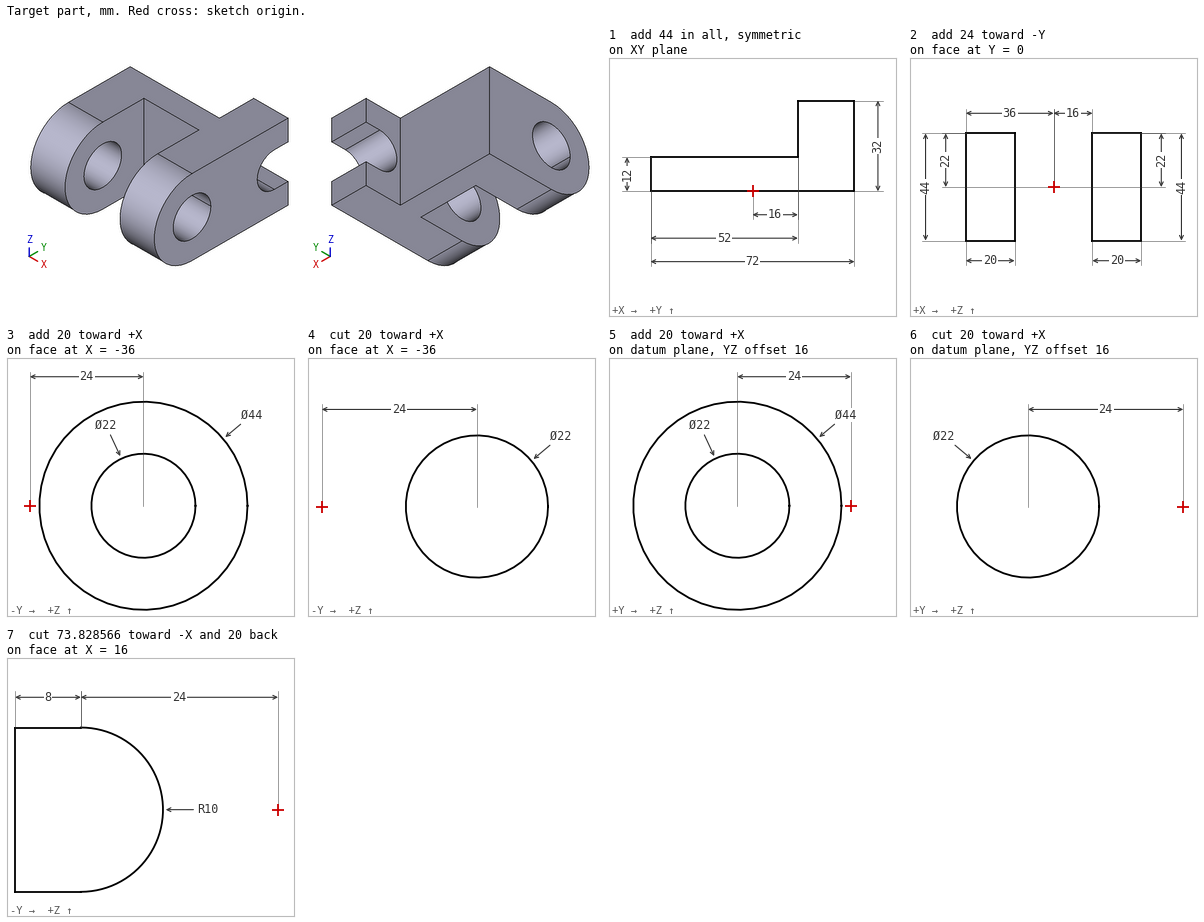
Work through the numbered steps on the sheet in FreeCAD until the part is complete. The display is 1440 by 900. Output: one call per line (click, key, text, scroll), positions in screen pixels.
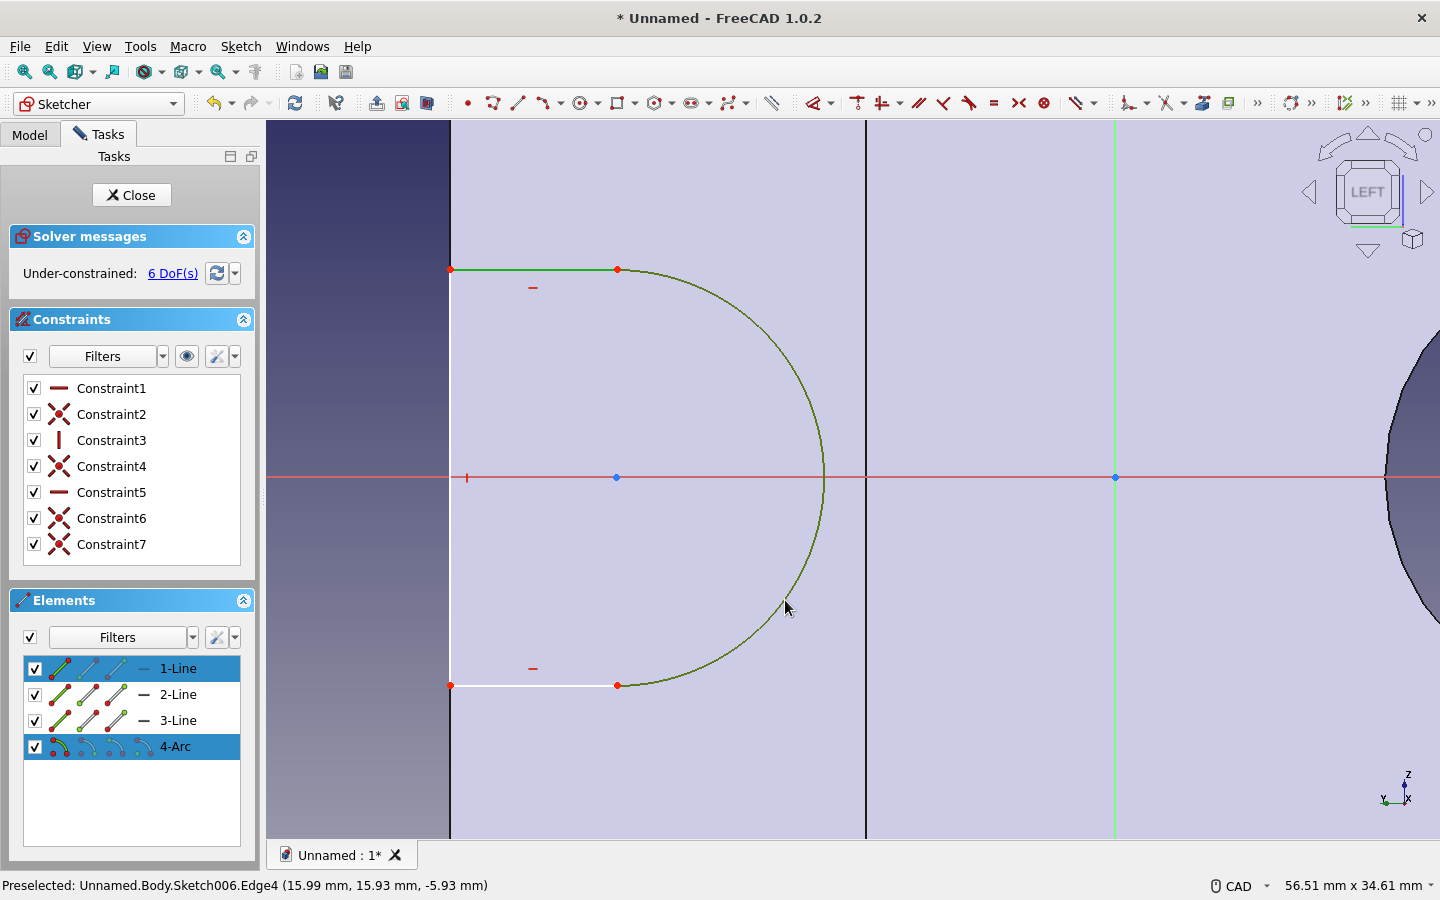
click(969, 104)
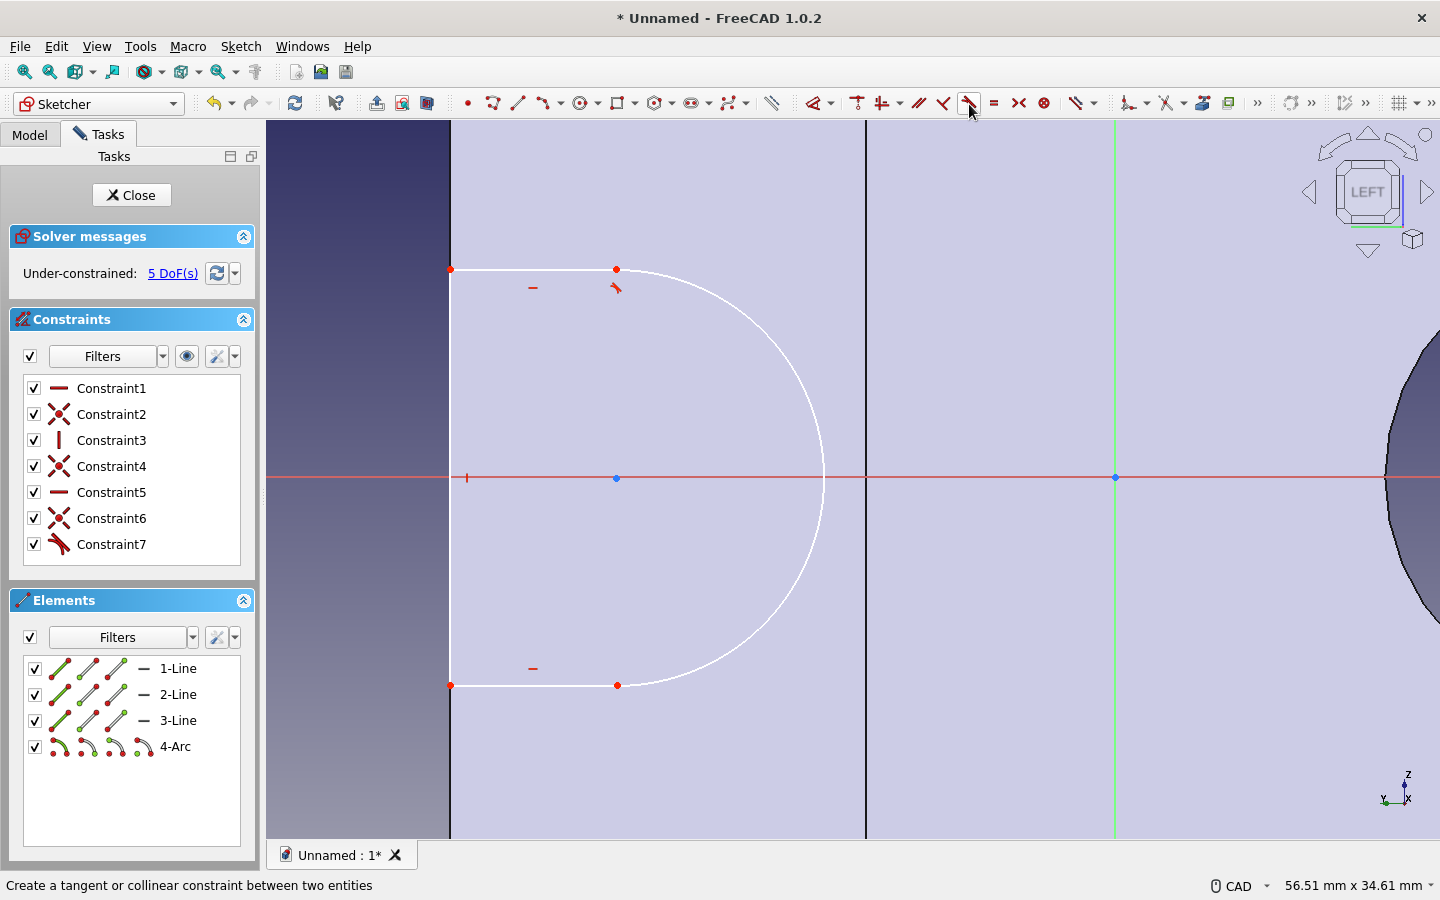
click(500, 686)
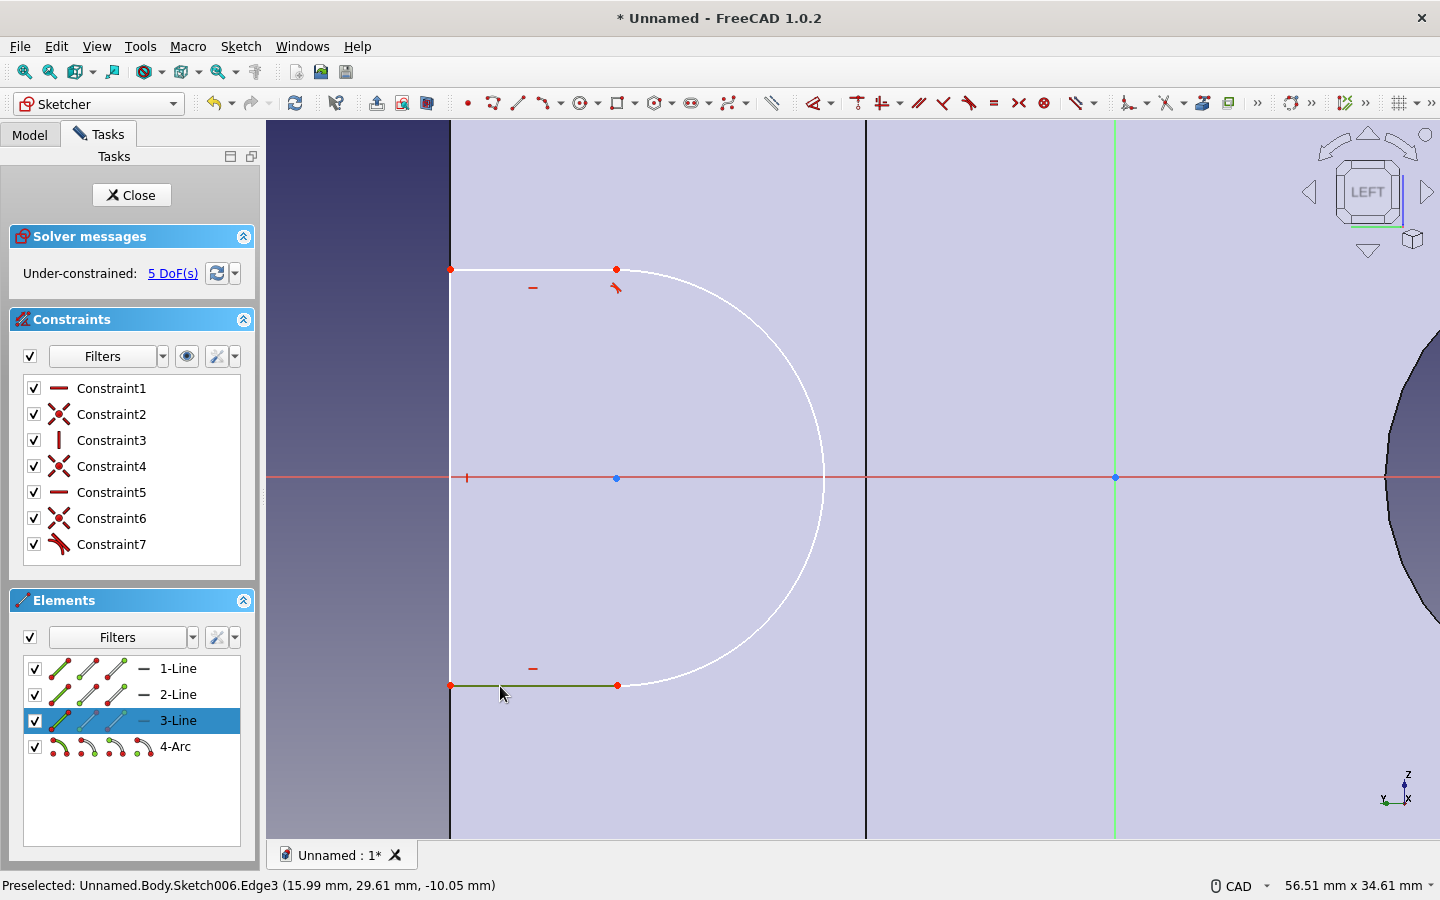
click(785, 600)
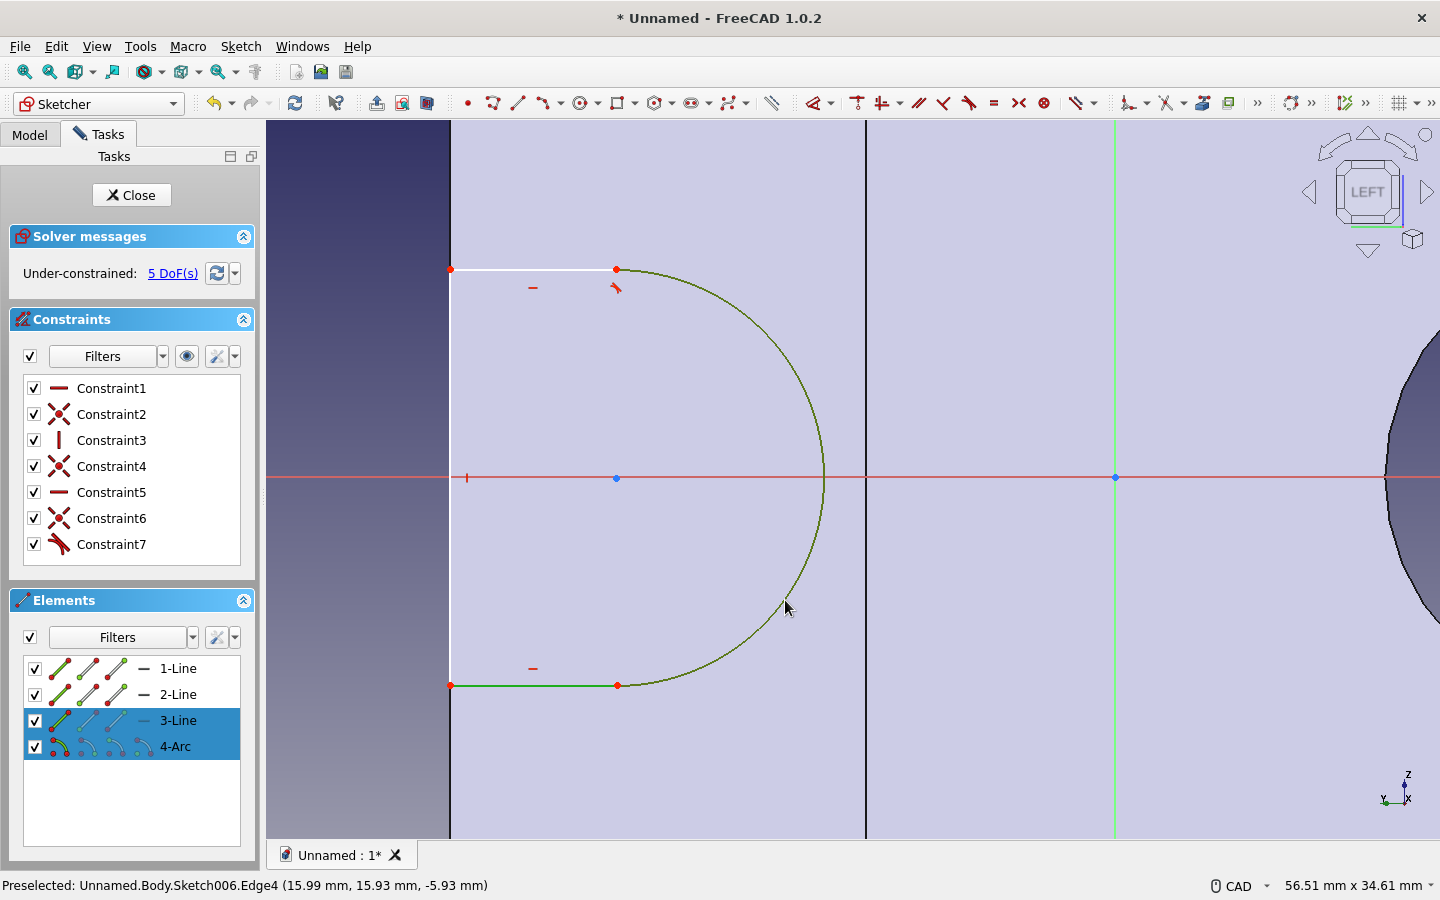
click(969, 104)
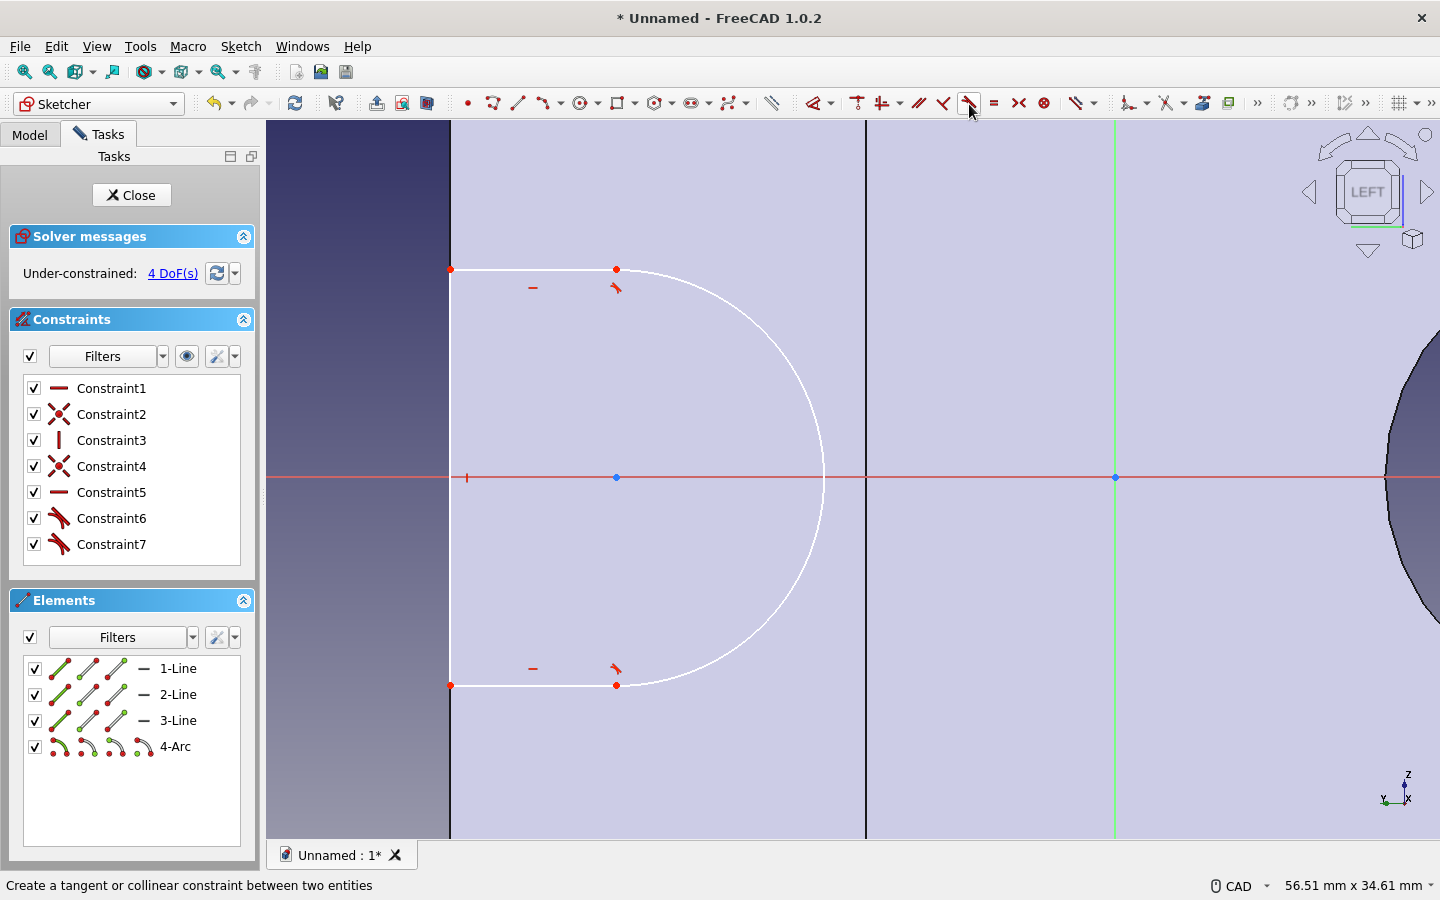
click(616, 478)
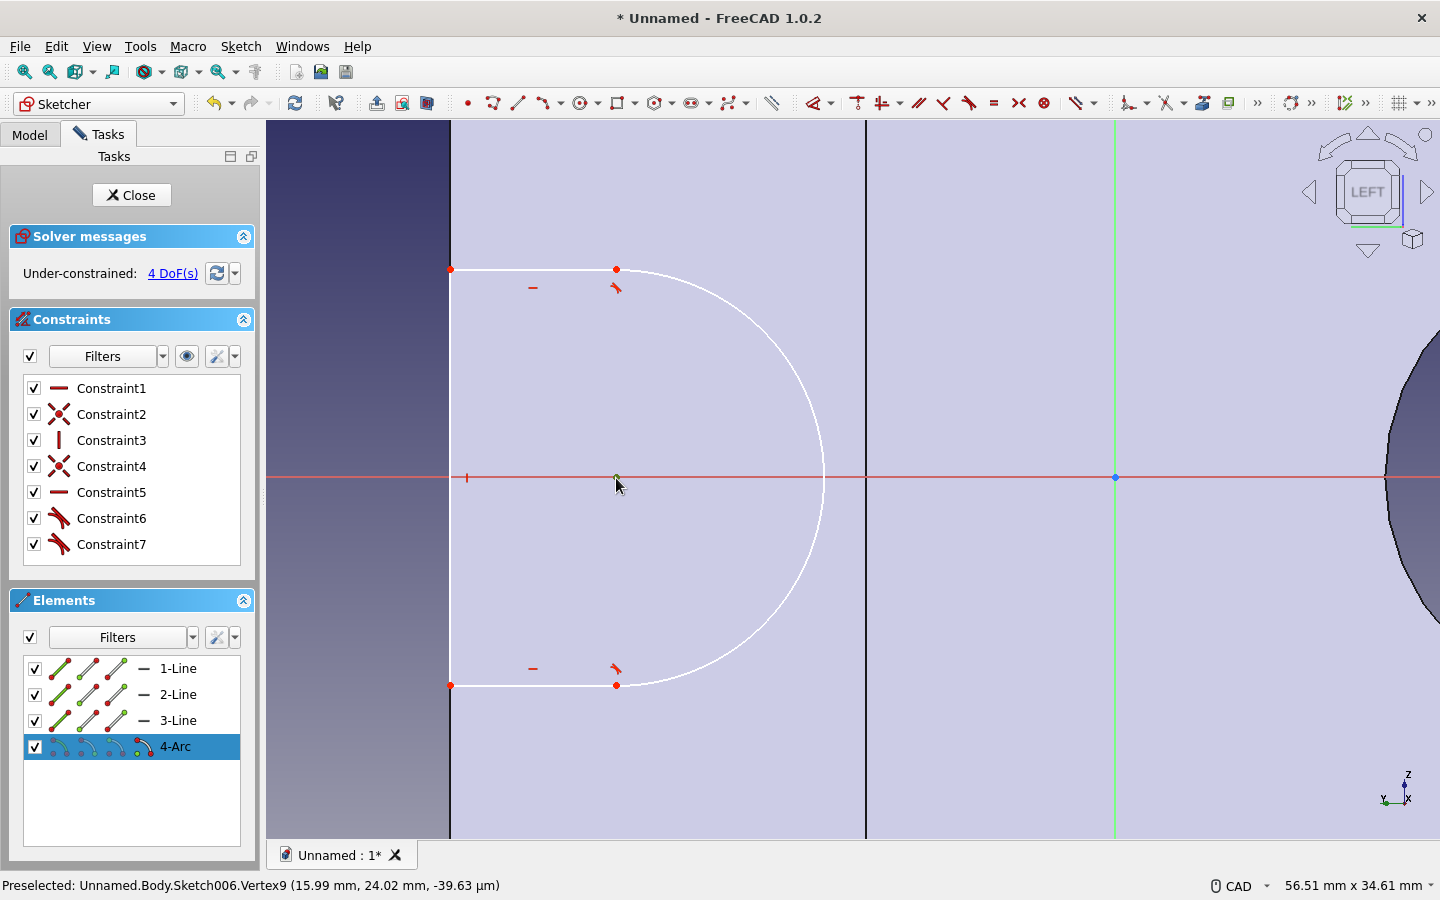
click(364, 477)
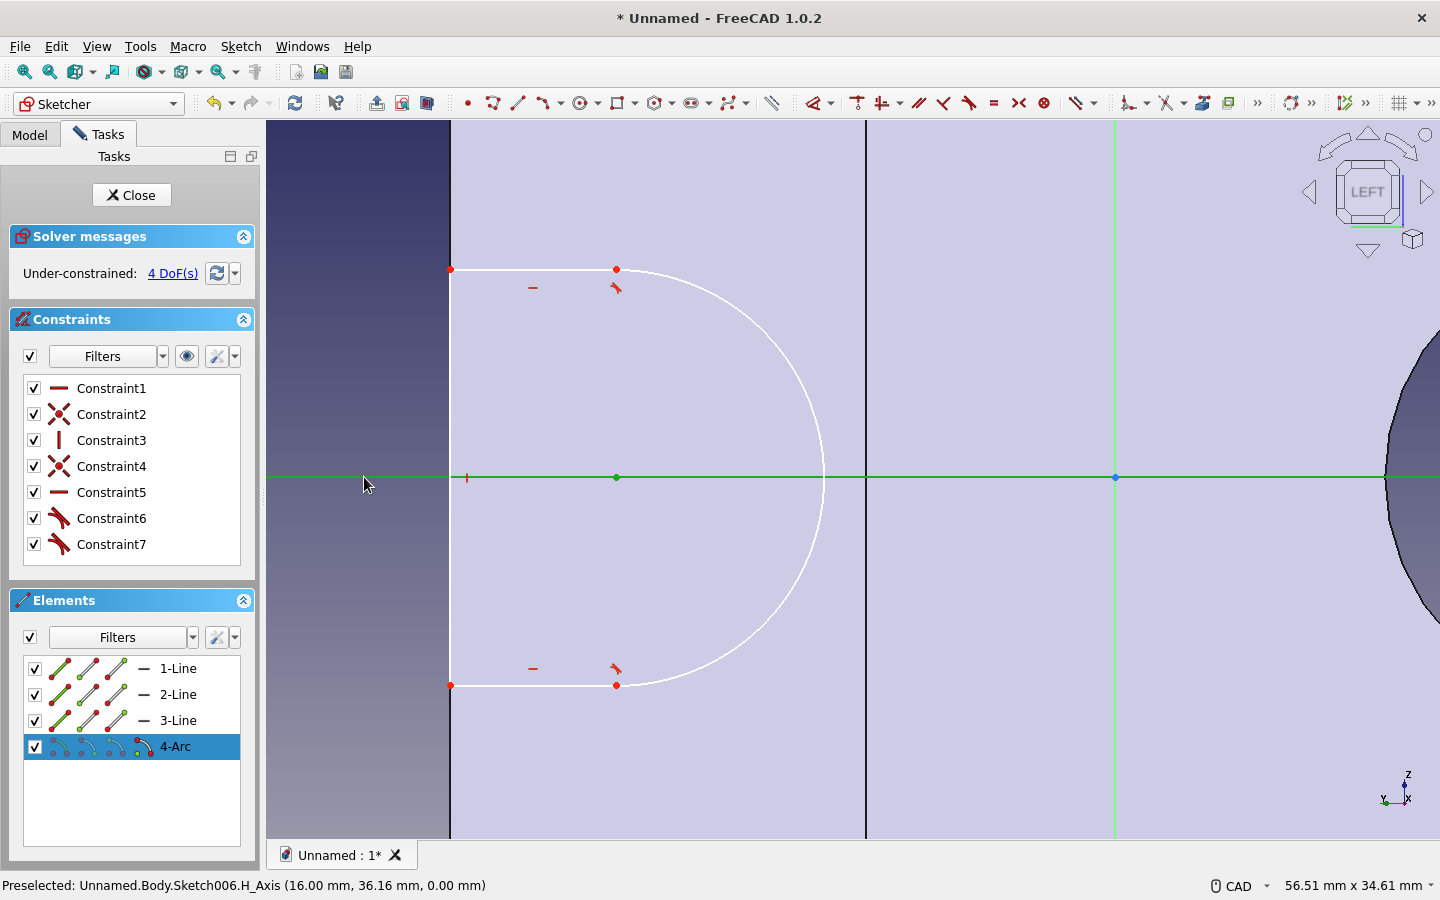
click(857, 104)